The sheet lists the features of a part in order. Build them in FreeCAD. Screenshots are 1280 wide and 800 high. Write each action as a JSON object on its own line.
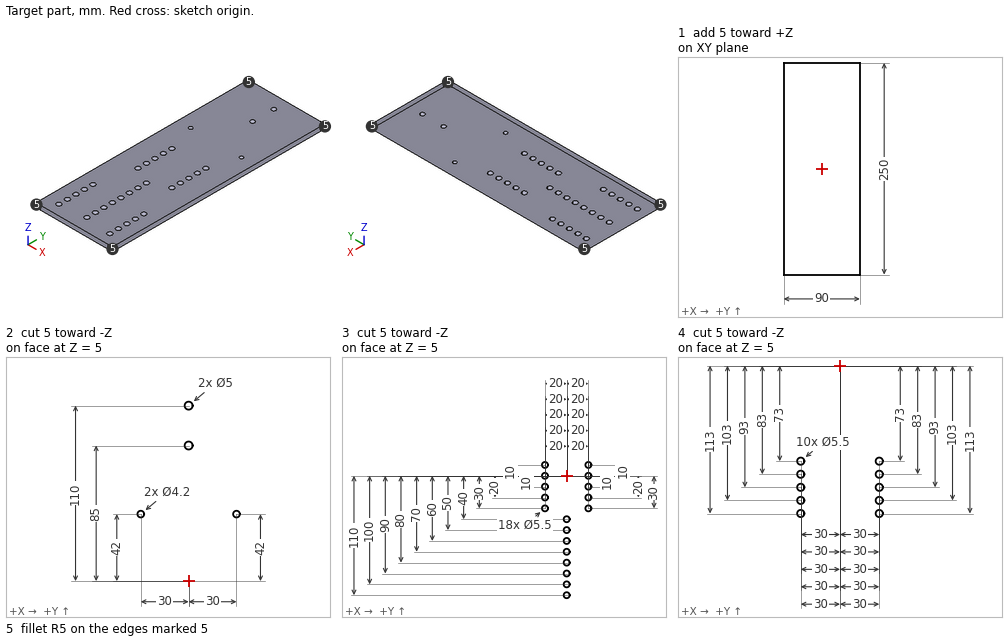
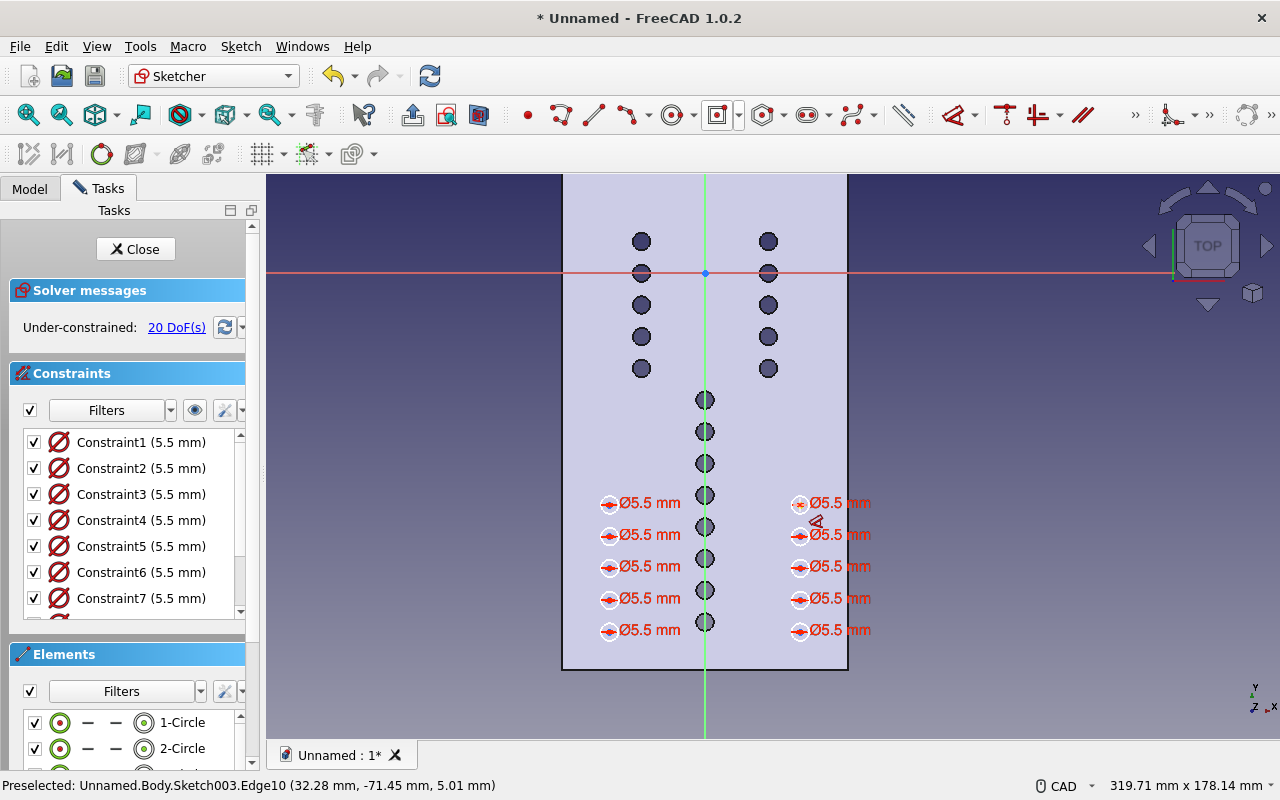
{"action": "left_click", "coordinate": [610, 632]}
{"action": "left_click", "coordinate": [657, 239]}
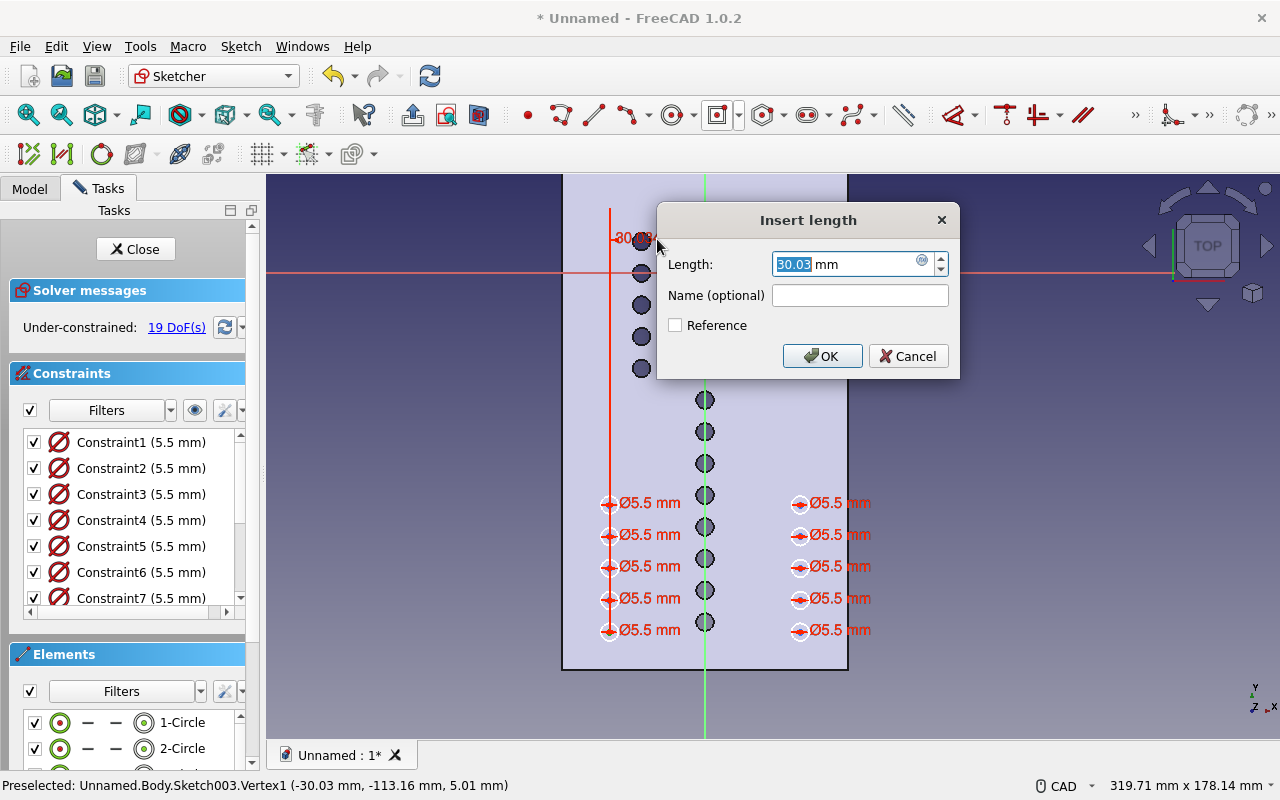
{"action": "type", "text": "30"}
{"action": "key", "text": "Return"}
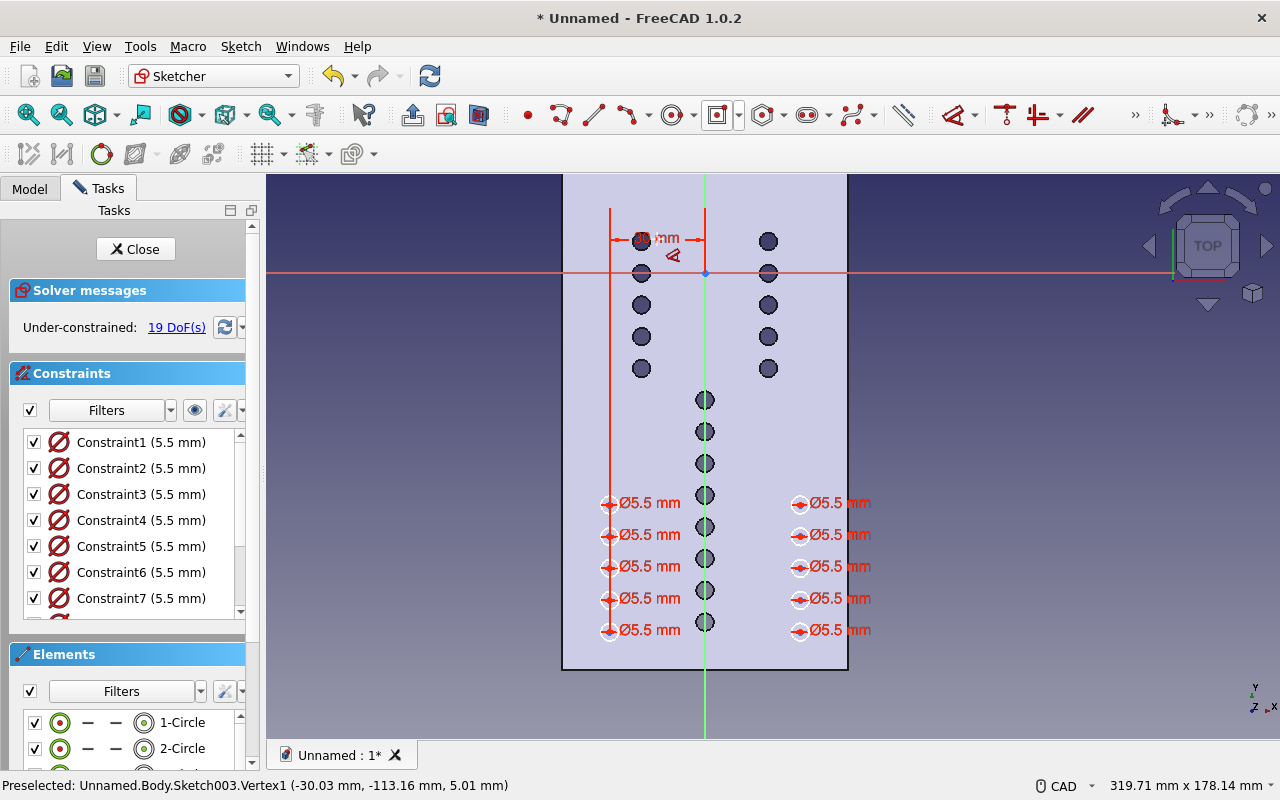
{"action": "left_click", "coordinate": [800, 632]}
{"action": "left_click", "coordinate": [753, 239]}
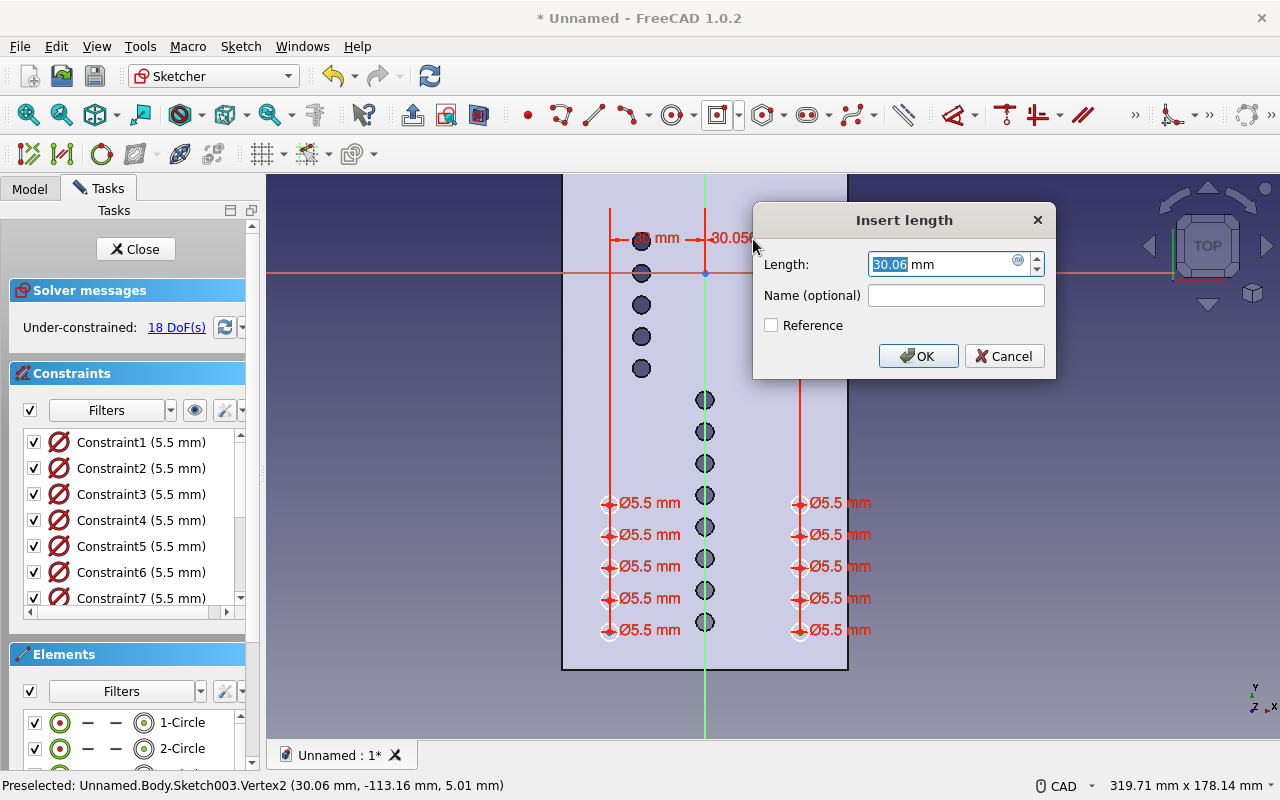
{"action": "type", "text": "30"}
{"action": "key", "text": "Return"}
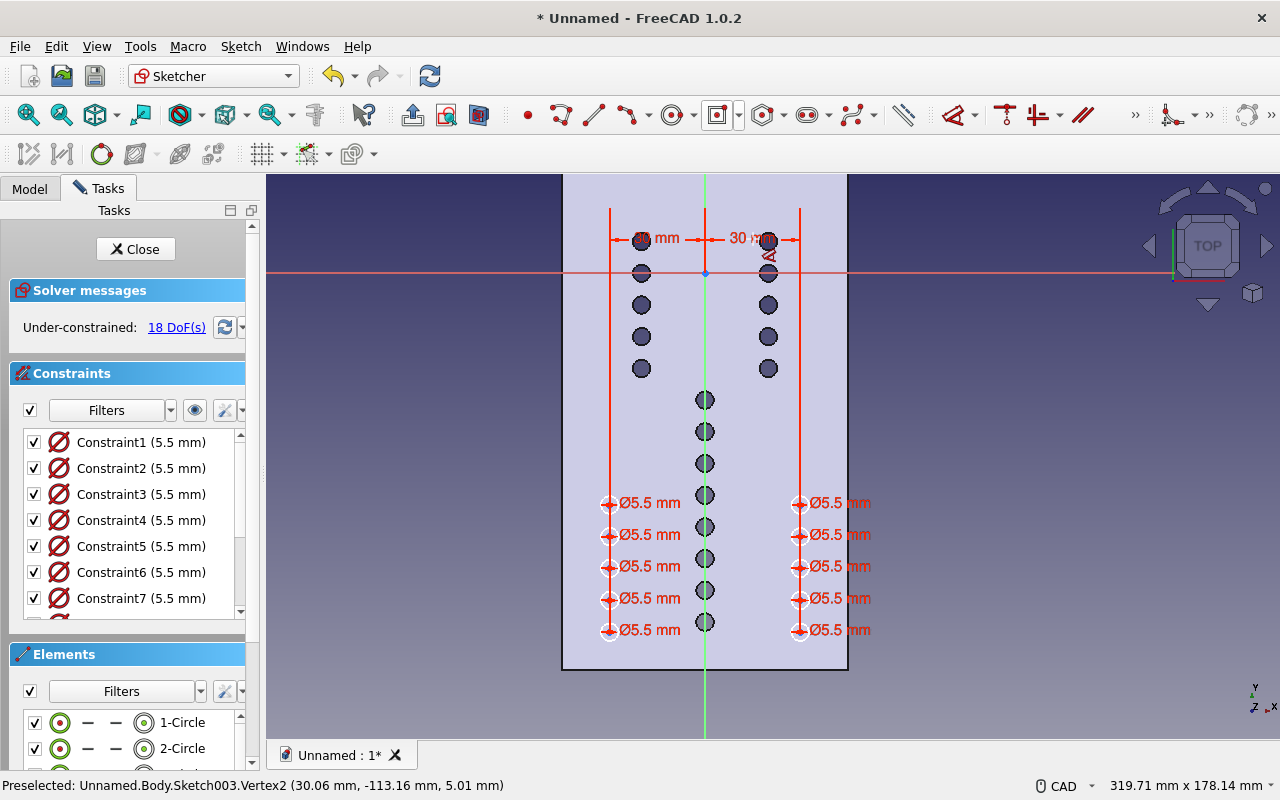
{"action": "left_click", "coordinate": [610, 600]}
{"action": "left_click", "coordinate": [657, 634]}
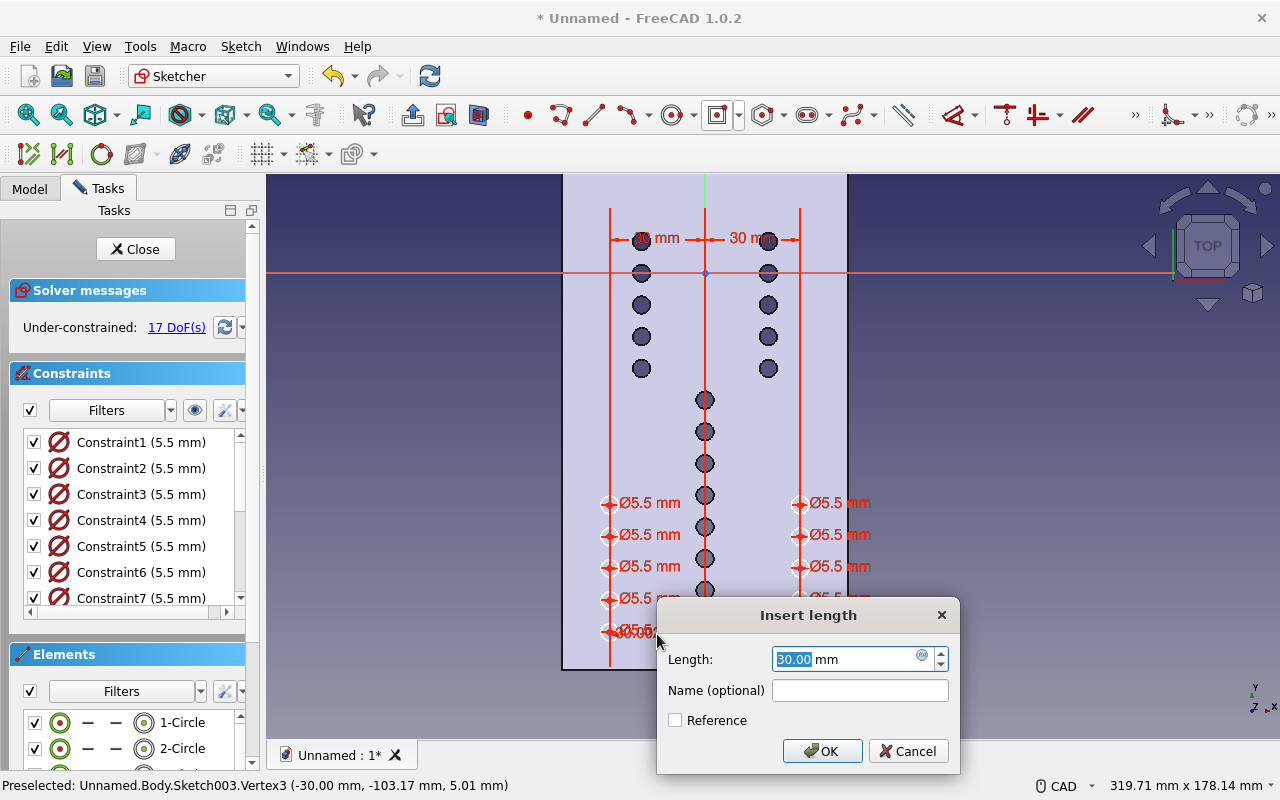
{"action": "type", "text": "30"}
{"action": "key", "text": "Return"}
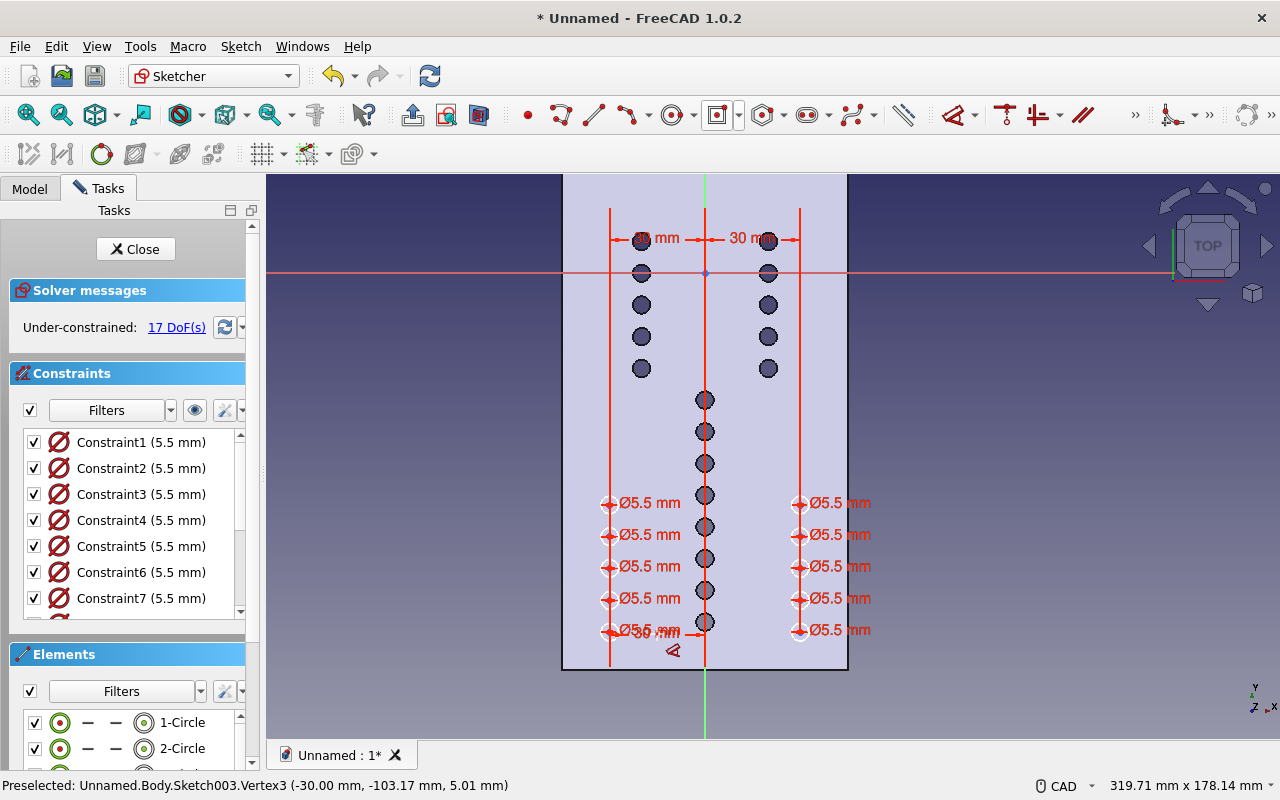
{"action": "left_click", "coordinate": [800, 600]}
{"action": "left_click", "coordinate": [753, 634]}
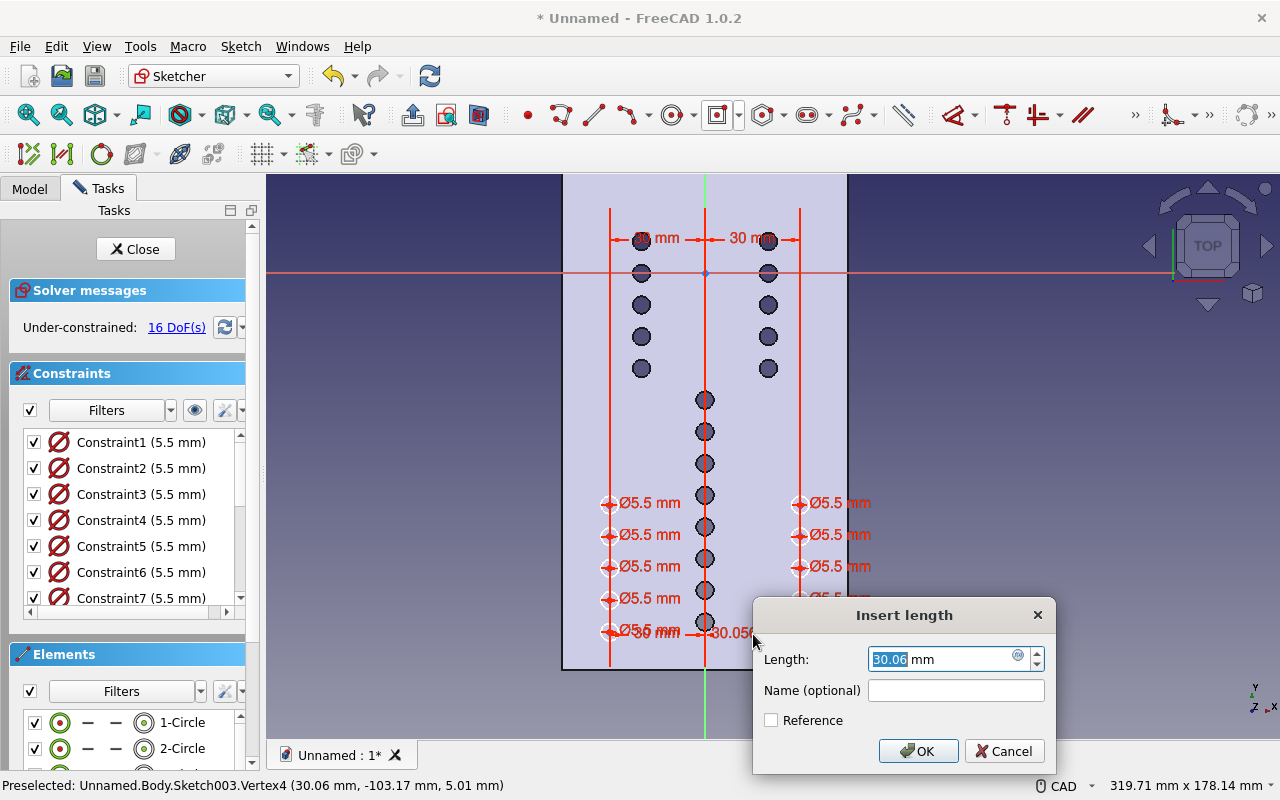
{"action": "type", "text": "30"}
{"action": "key", "text": "Return"}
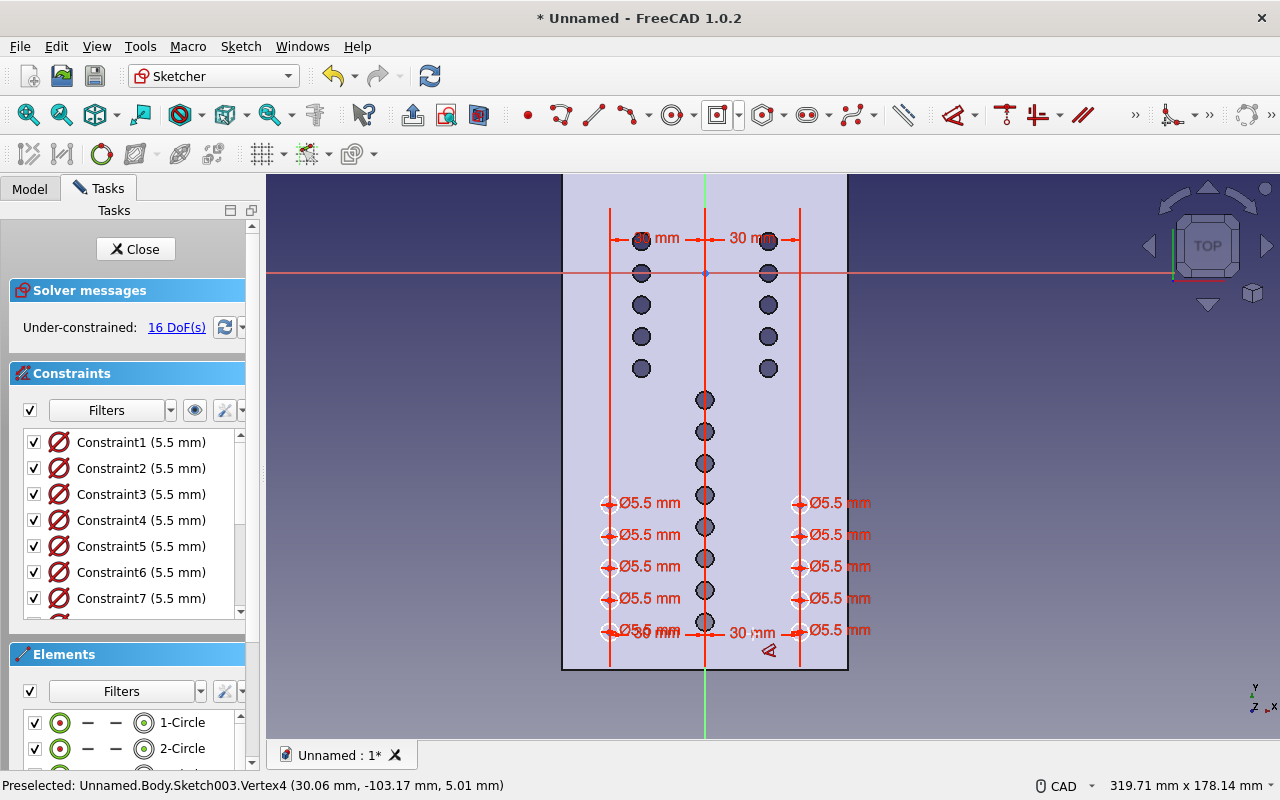
{"action": "left_click", "coordinate": [610, 568]}
{"action": "left_click", "coordinate": [657, 602]}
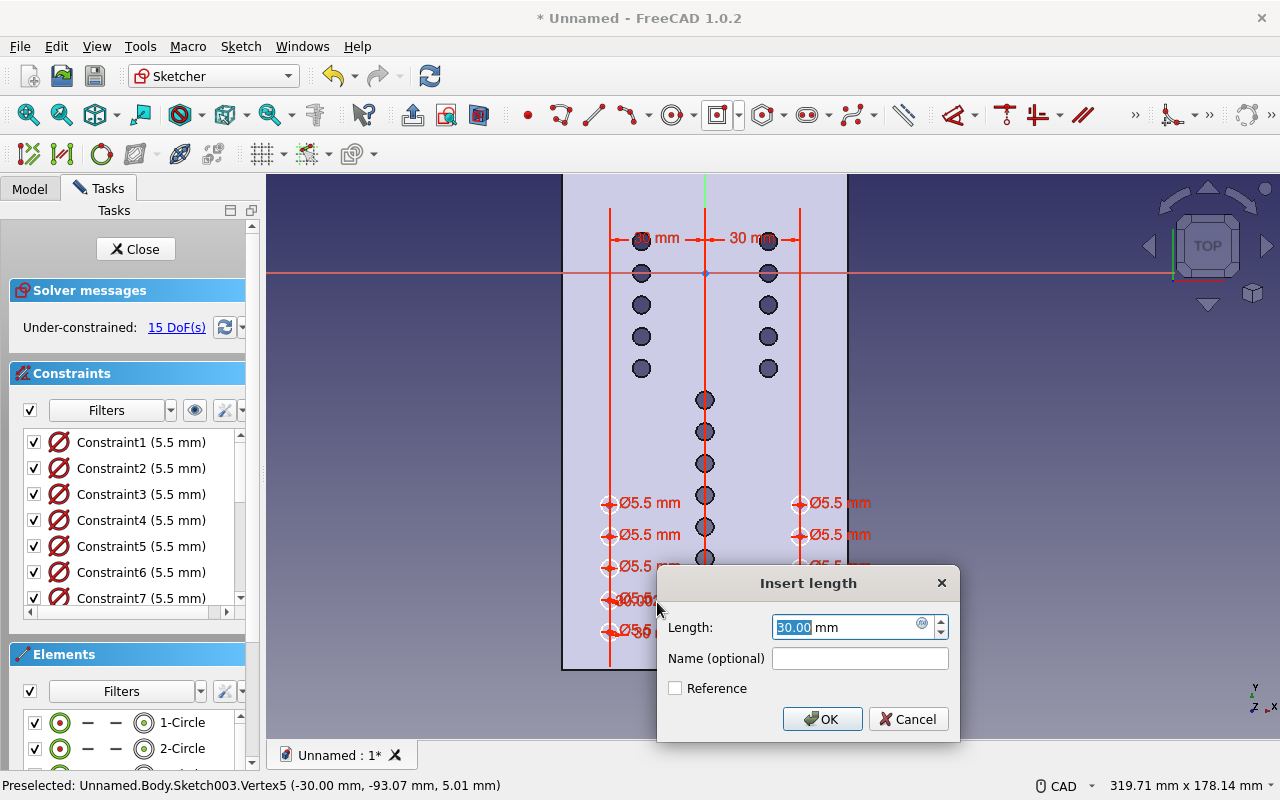
{"action": "type", "text": "30"}
{"action": "key", "text": "Return"}